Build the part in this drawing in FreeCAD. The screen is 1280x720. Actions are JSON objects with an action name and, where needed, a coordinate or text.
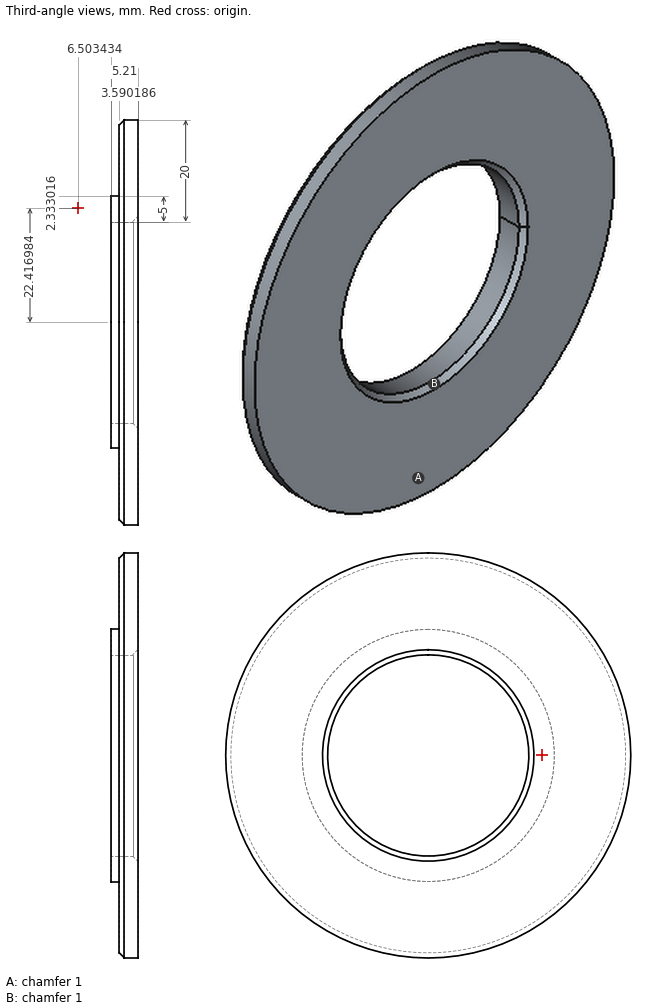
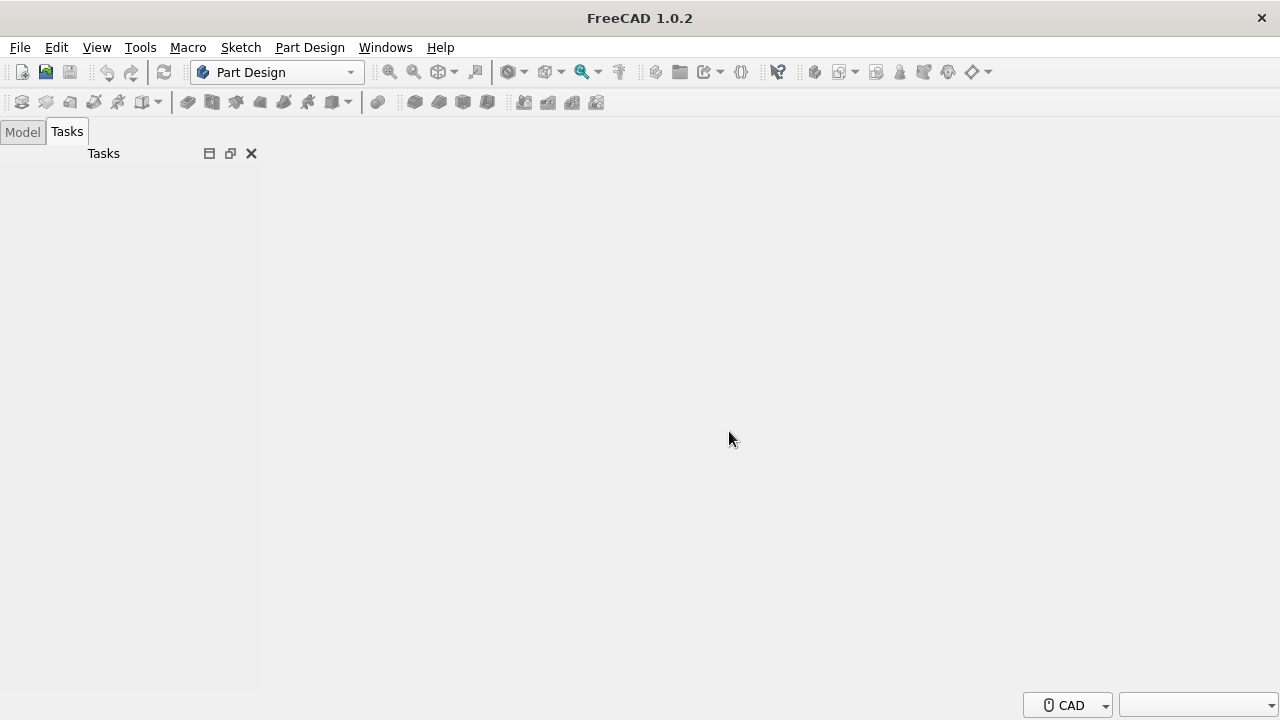
{"action": "key", "text": "ctrl+n"}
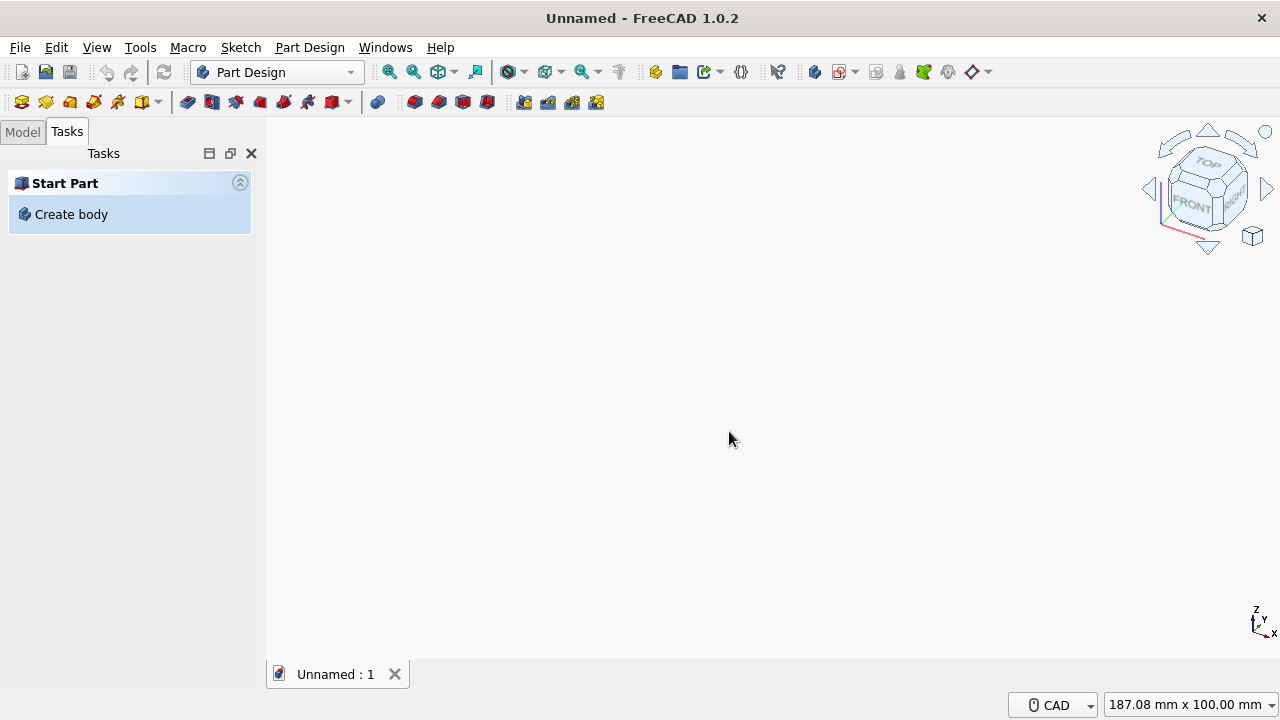
{"action": "left_click", "coordinate": [840, 72]}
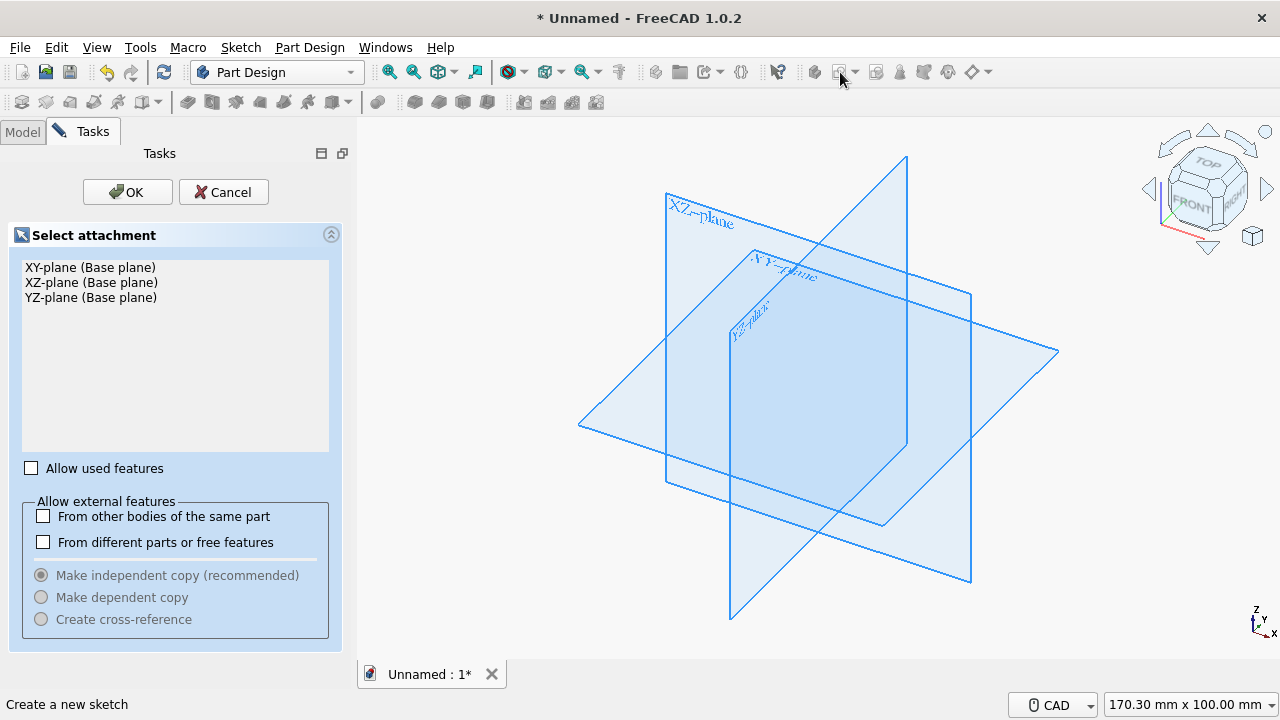
{"action": "left_click", "coordinate": [82, 268]}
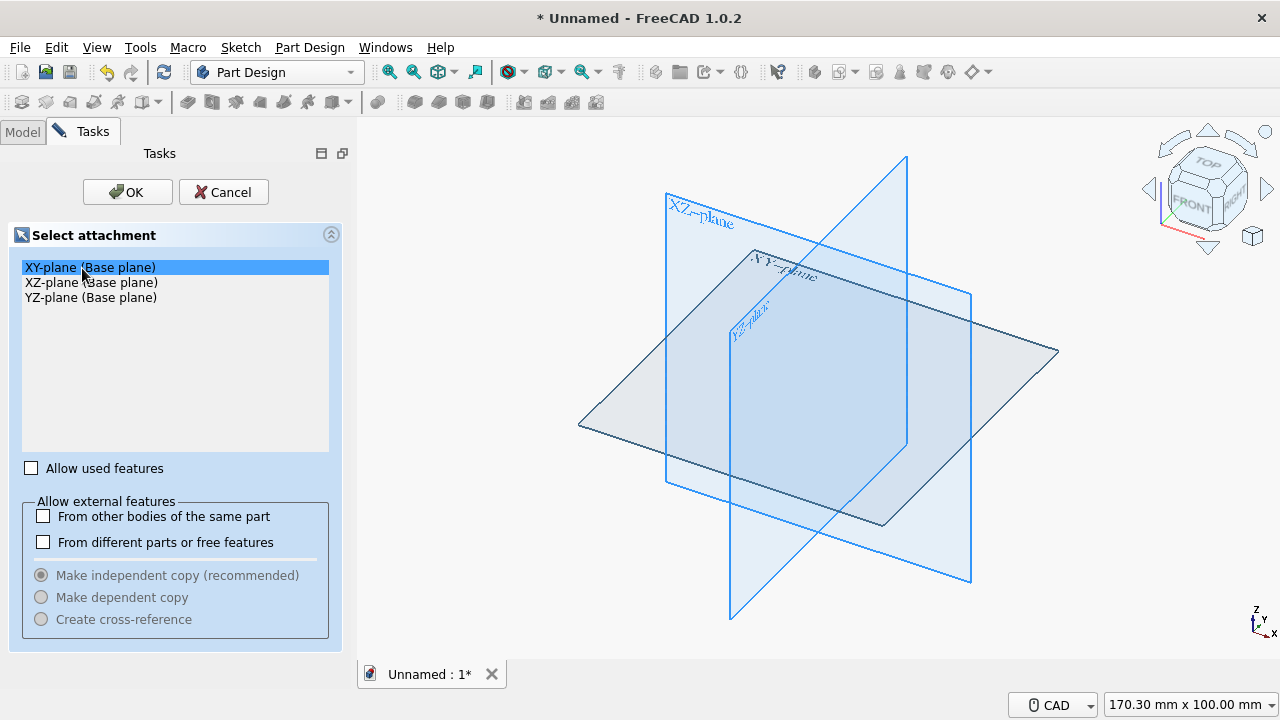
{"action": "left_click", "coordinate": [128, 192]}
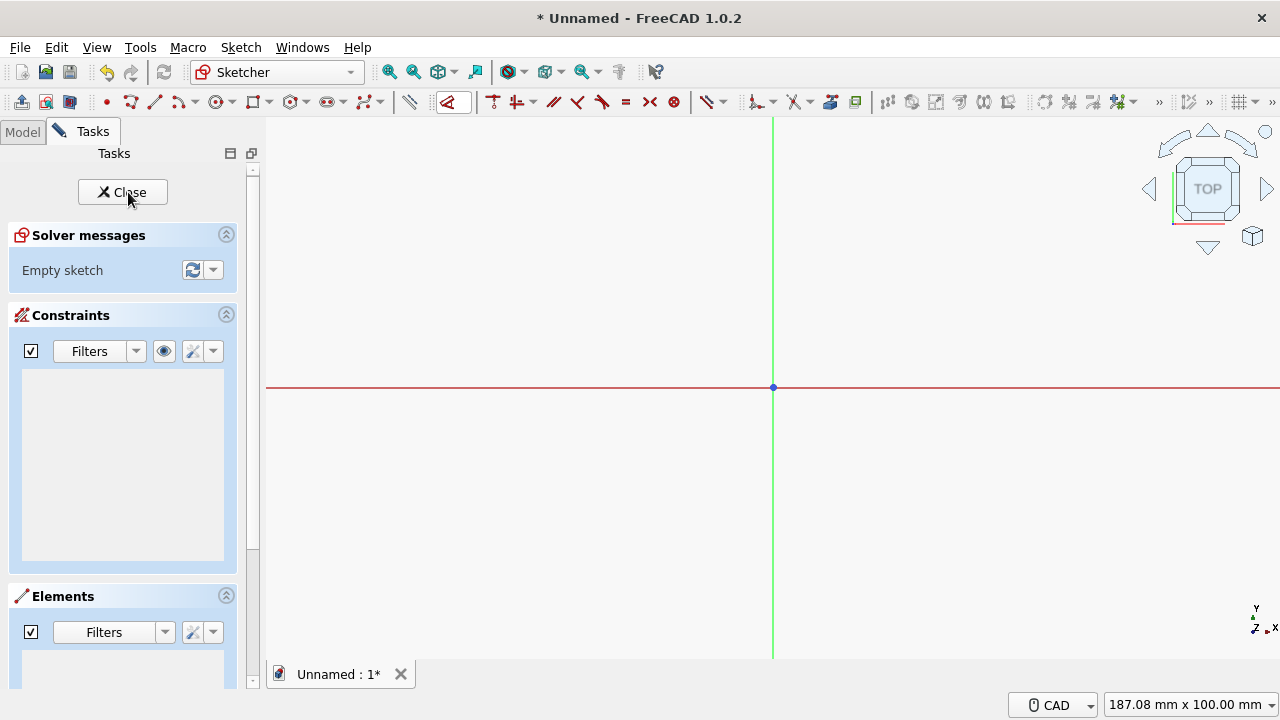
{"action": "scroll", "coordinate": [1015, 430], "scroll_direction": "up", "scroll_amount": 2}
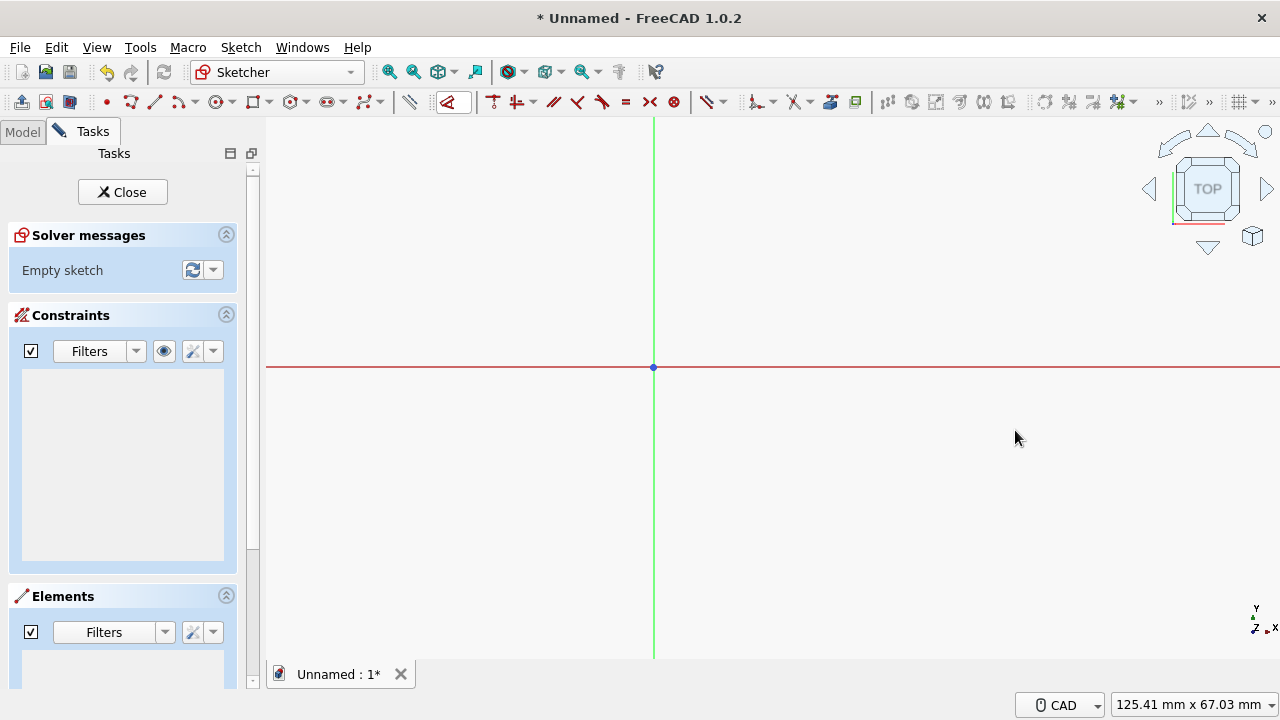
{"action": "key", "text": "g m"}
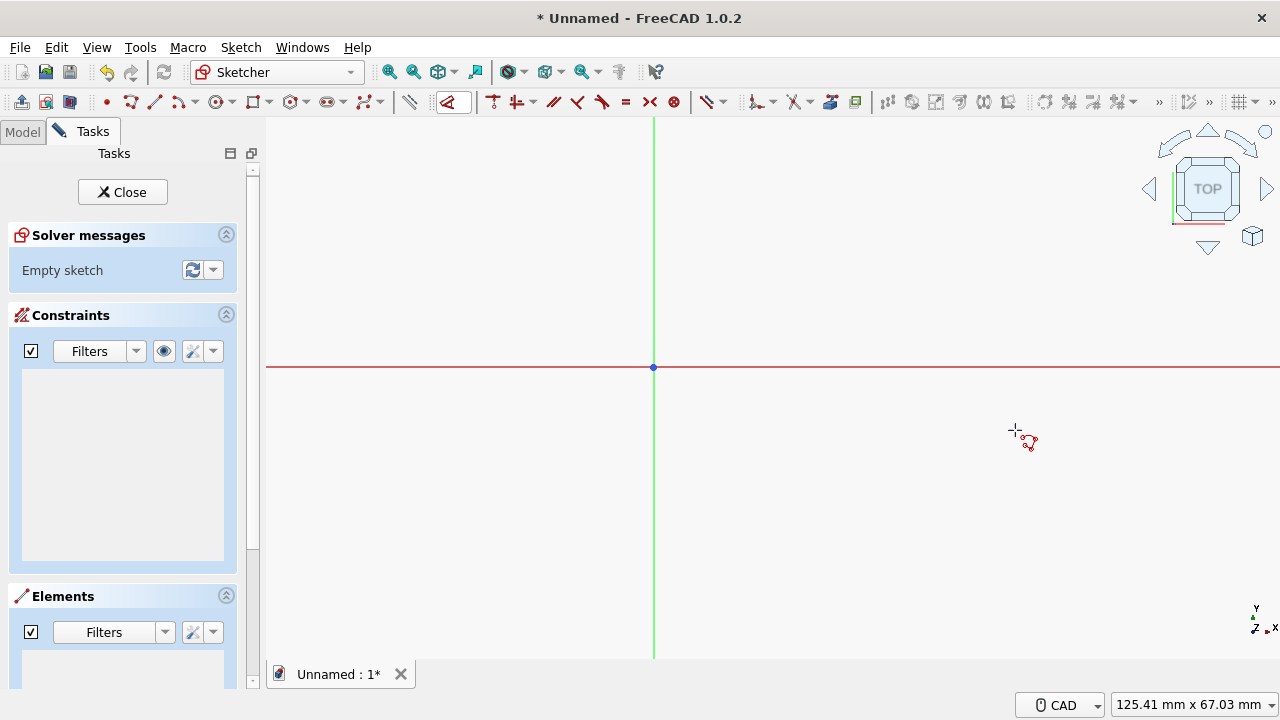
{"action": "left_click", "coordinate": [706, 348]}
{"action": "left_click", "coordinate": [706, 389]}
{"action": "left_click", "coordinate": [748, 389]}
{"action": "left_click", "coordinate": [748, 227]}
{"action": "left_click", "coordinate": [719, 227]}
{"action": "left_click", "coordinate": [719, 348]}
{"action": "left_click", "coordinate": [706, 349]}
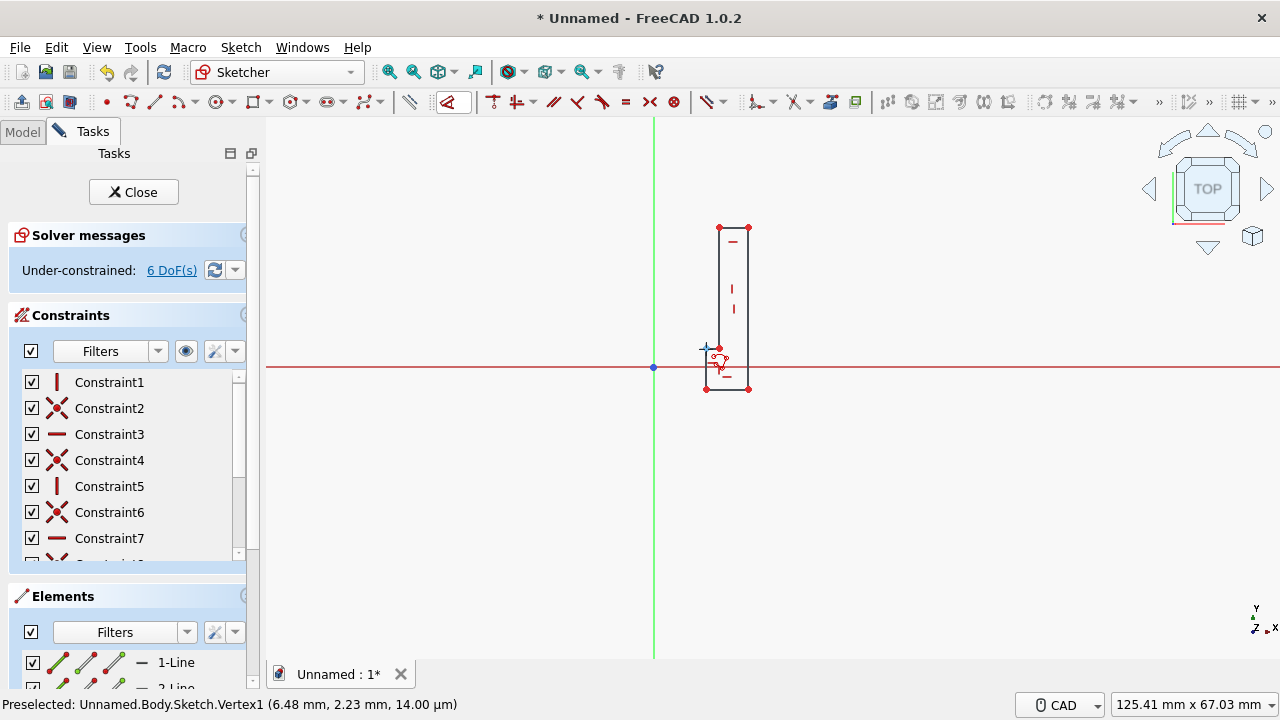
{"action": "key", "text": "g l"}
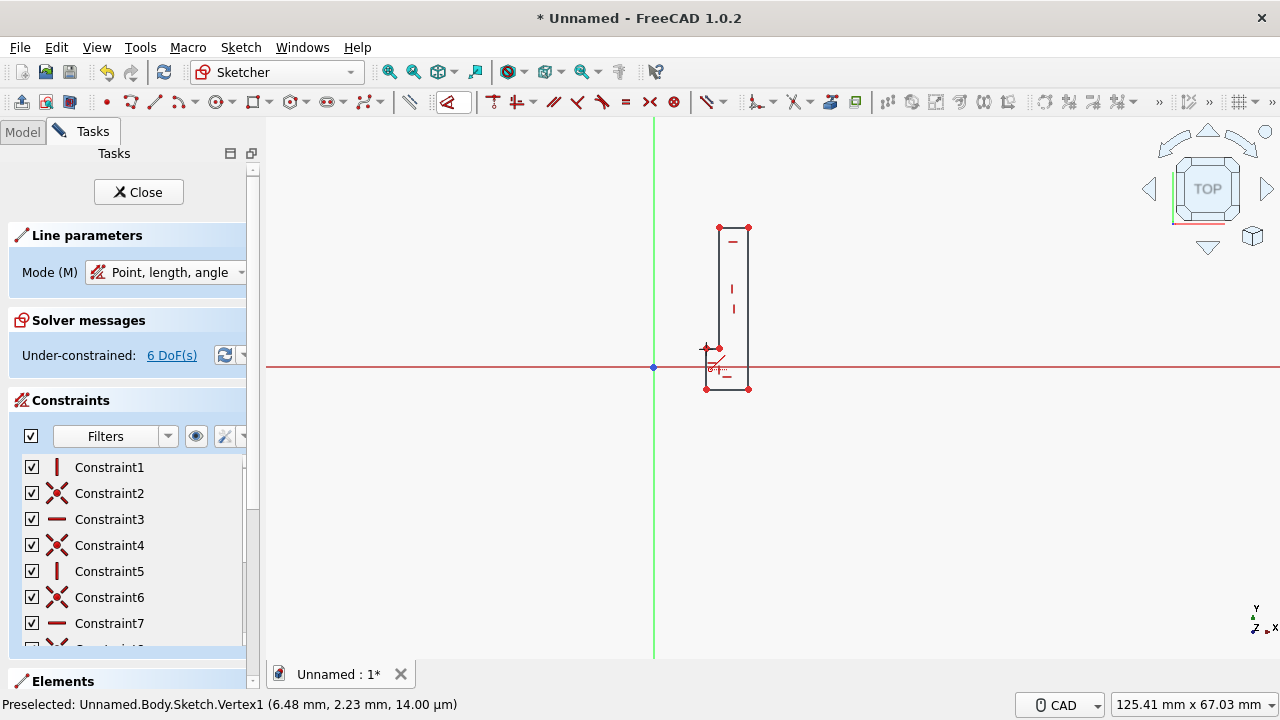
{"action": "left_click", "coordinate": [700, 548]}
{"action": "left_click", "coordinate": [755, 548]}
{"action": "key", "text": "Escape"}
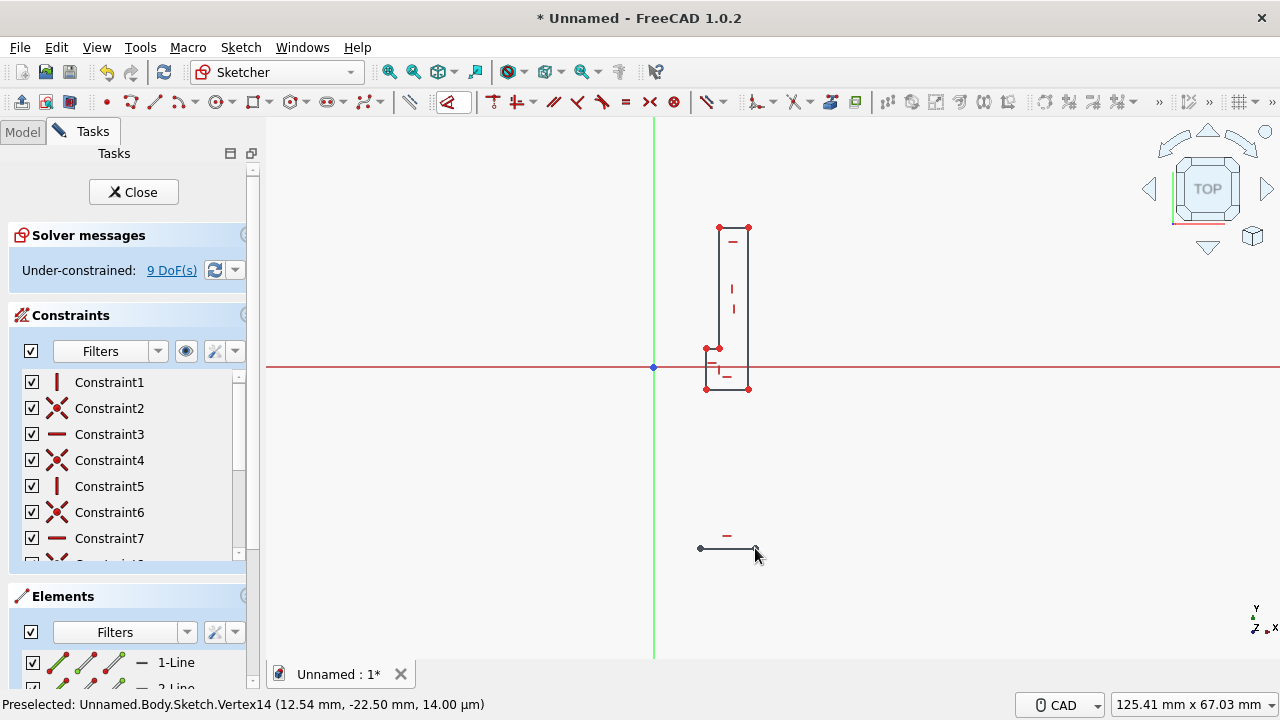
{"action": "left_click", "coordinate": [717, 549]}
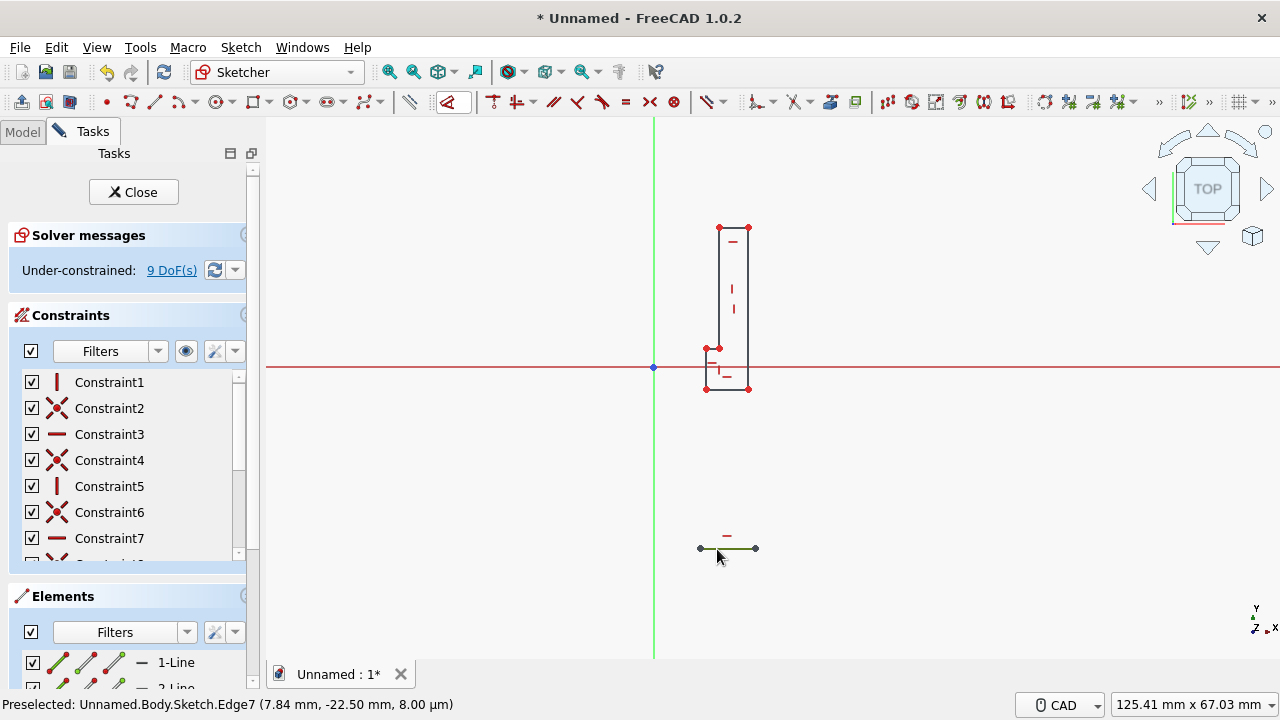
{"action": "key", "text": "g n"}